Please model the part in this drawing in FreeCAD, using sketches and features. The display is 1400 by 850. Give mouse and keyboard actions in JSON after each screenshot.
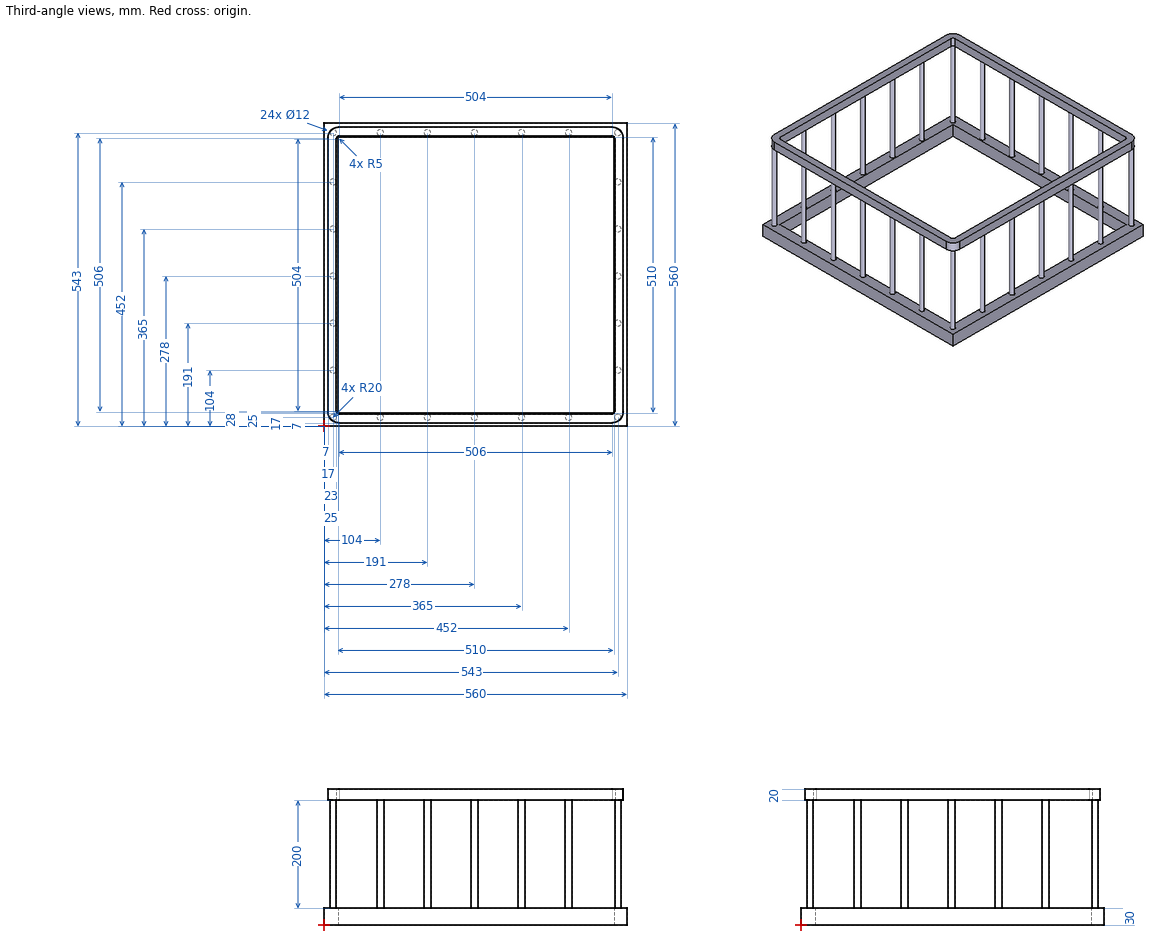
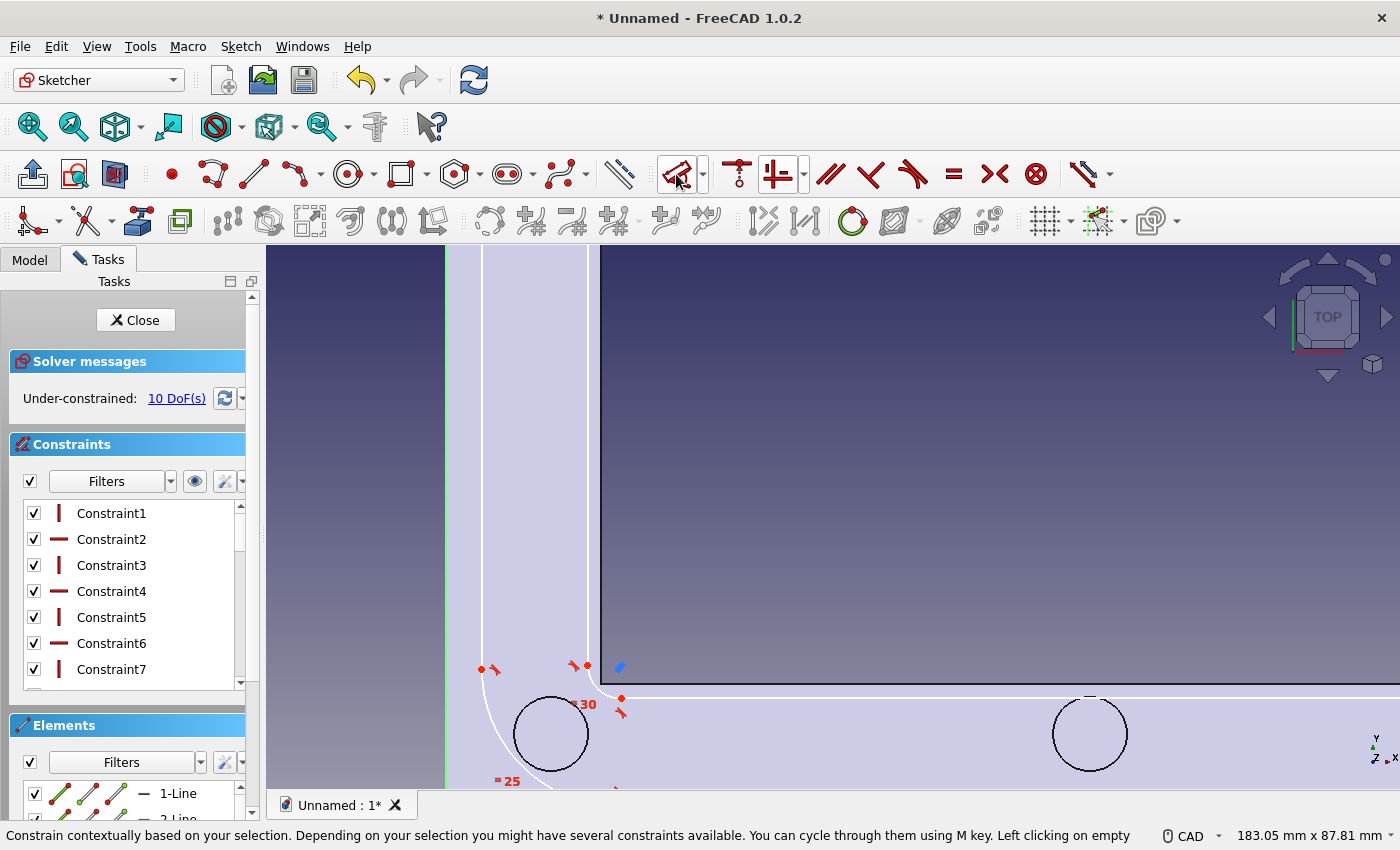
{"action": "scroll", "coordinate": [591, 690], "scroll_direction": "down", "scroll_amount": 11}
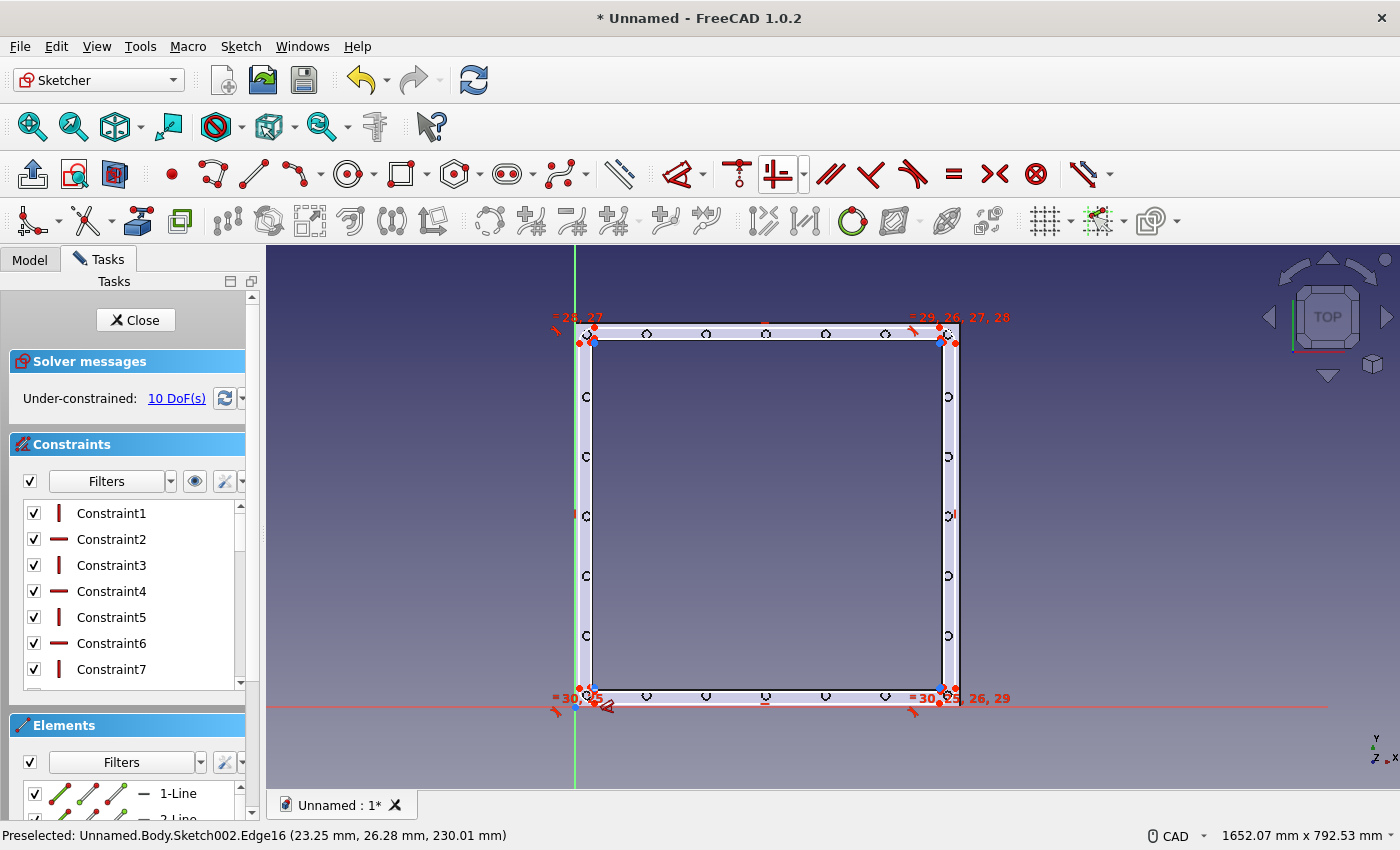
{"action": "scroll", "coordinate": [581, 695], "scroll_direction": "up", "scroll_amount": 6}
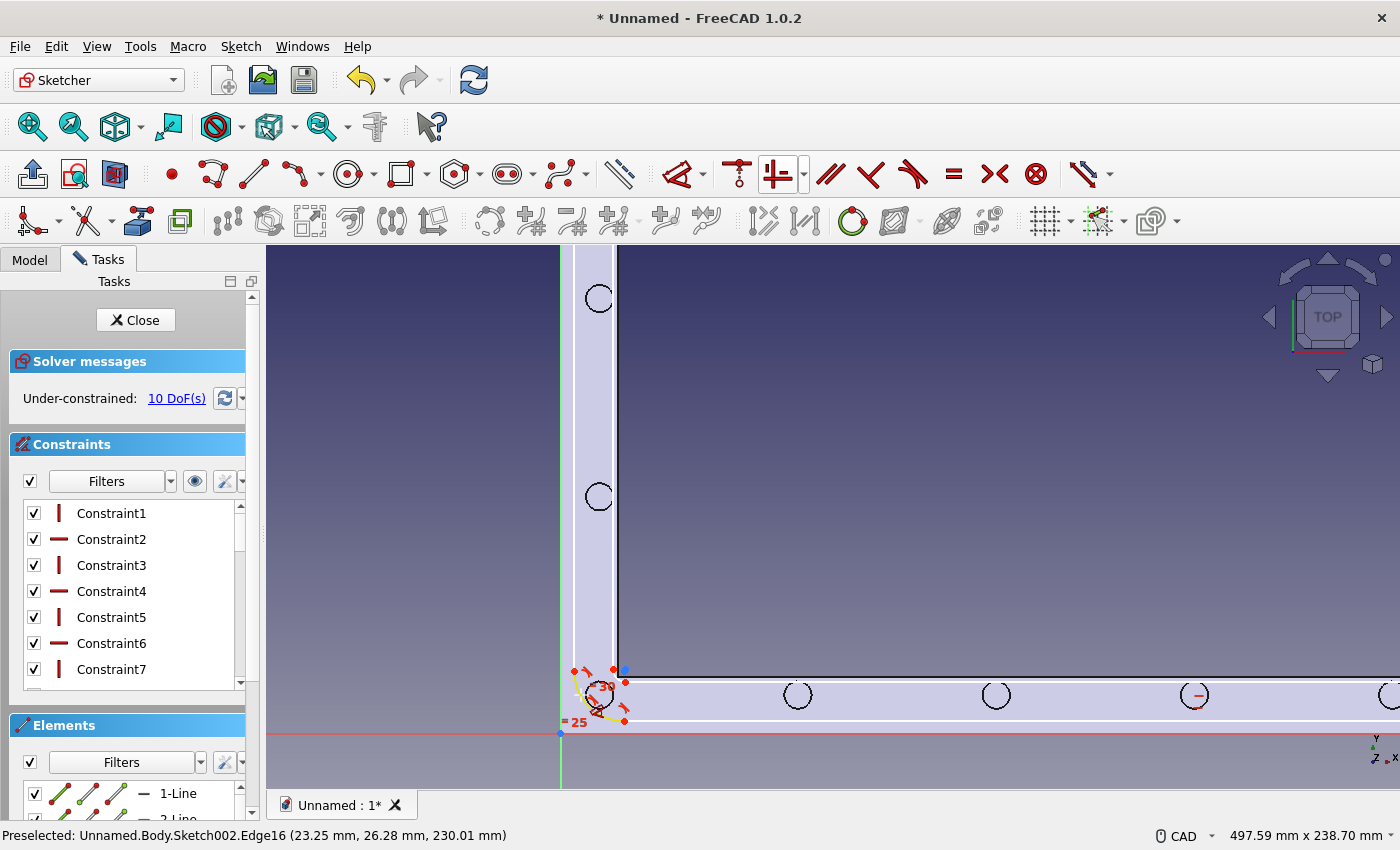
{"action": "left_click", "coordinate": [580, 694]}
{"action": "left_click", "coordinate": [543, 669]}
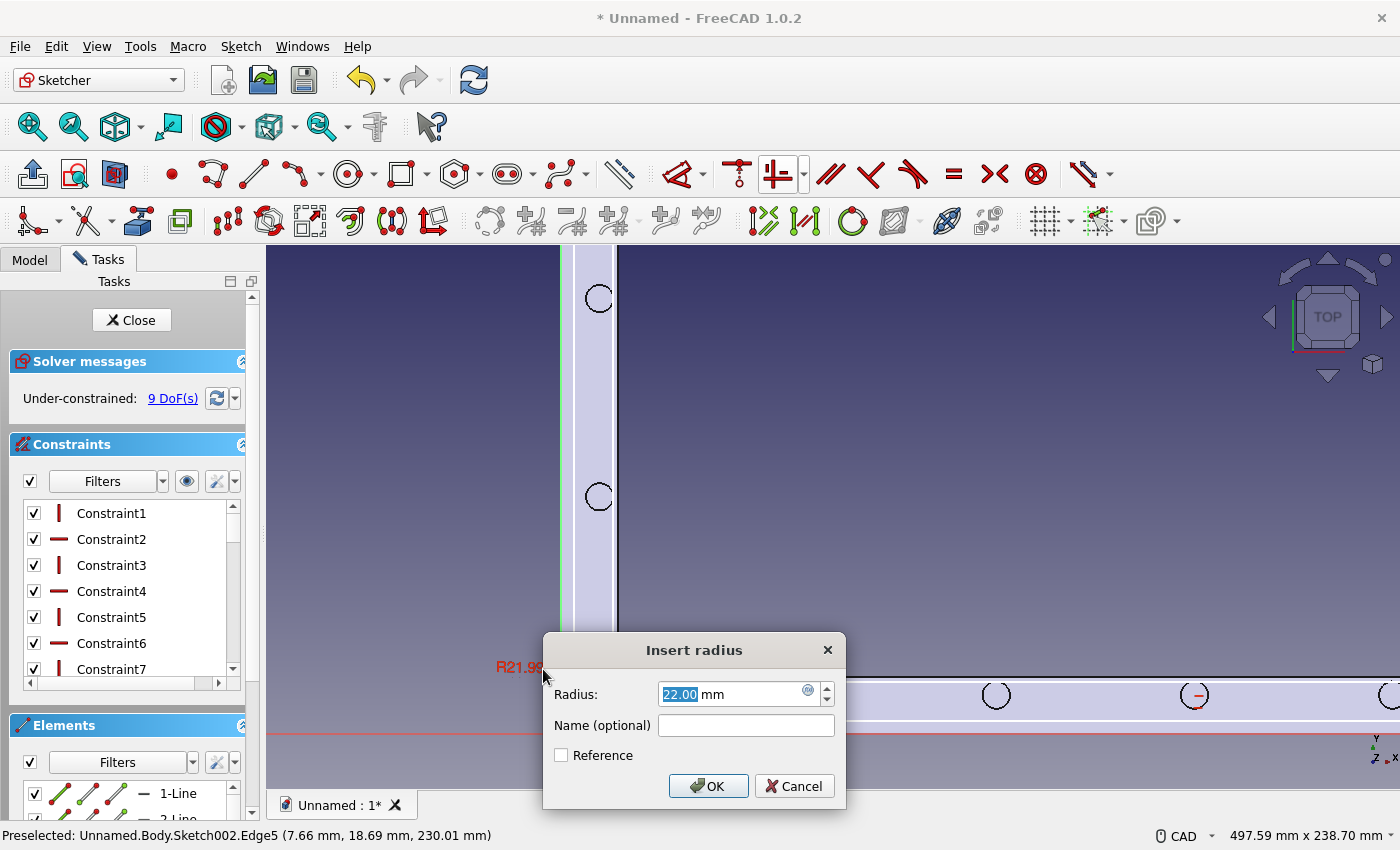
{"action": "type", "text": "20"}
{"action": "key", "text": "Return"}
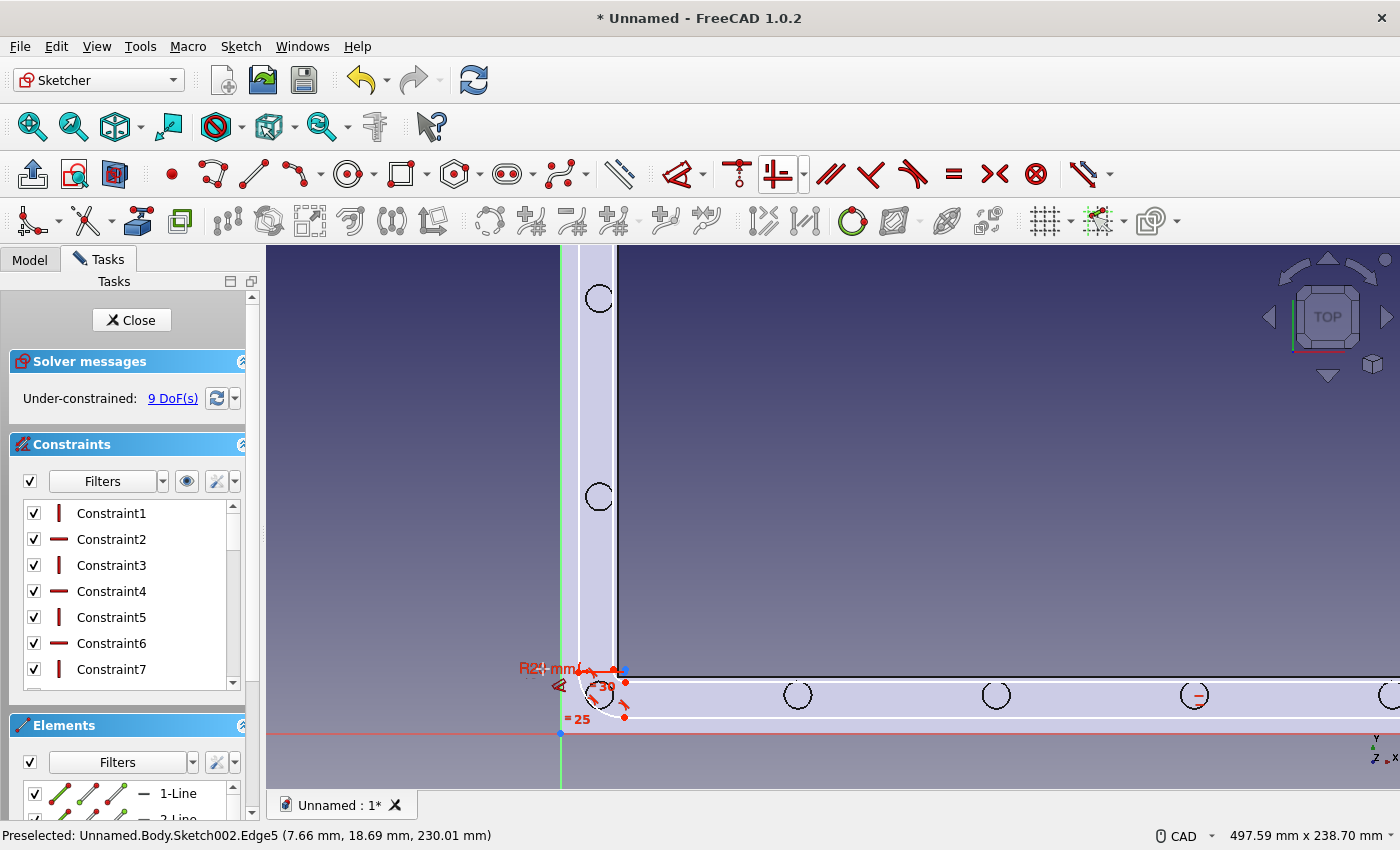
{"action": "scroll", "coordinate": [581, 695], "scroll_direction": "down", "scroll_amount": 6}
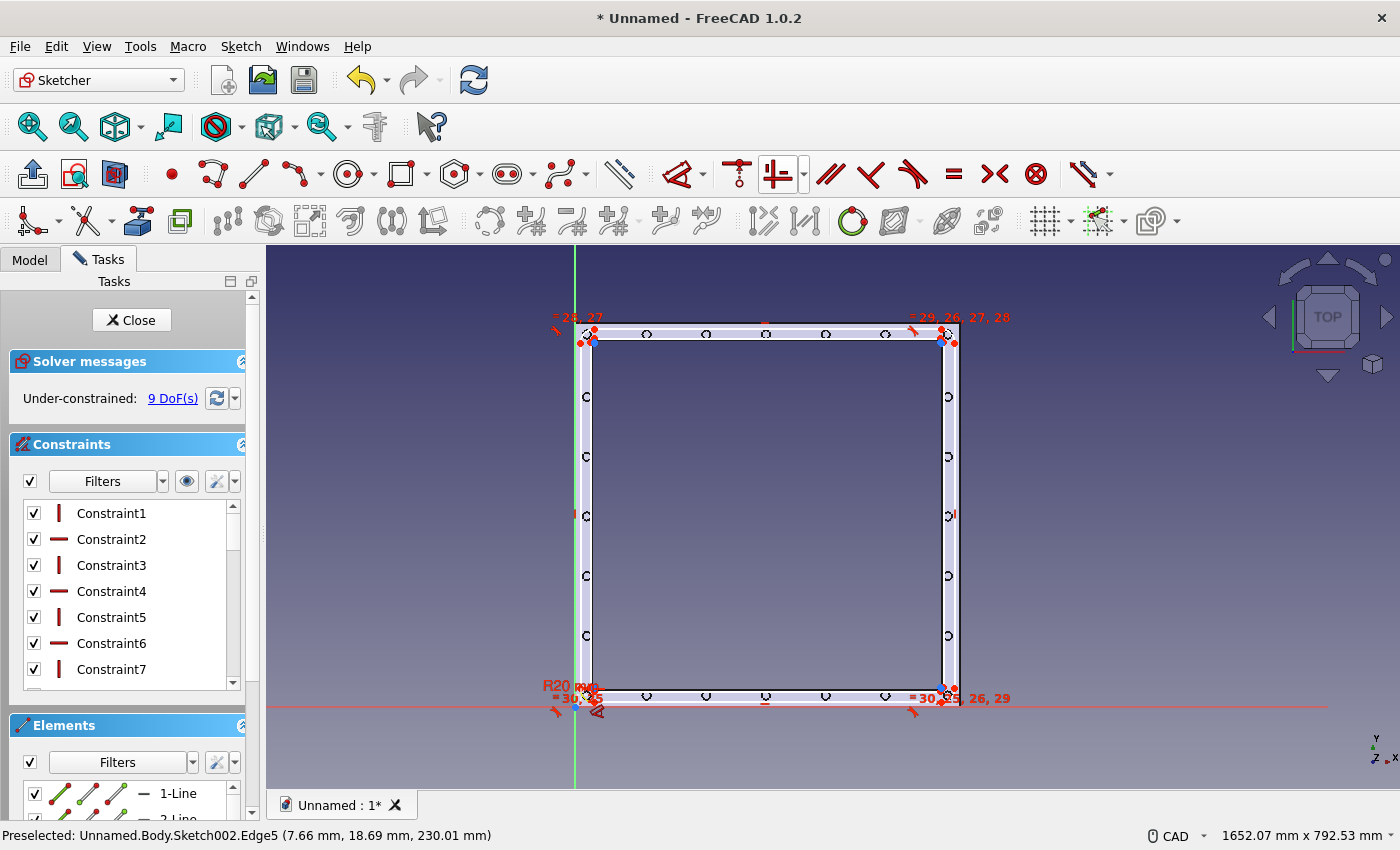
{"action": "scroll", "coordinate": [592, 340], "scroll_direction": "up", "scroll_amount": 13}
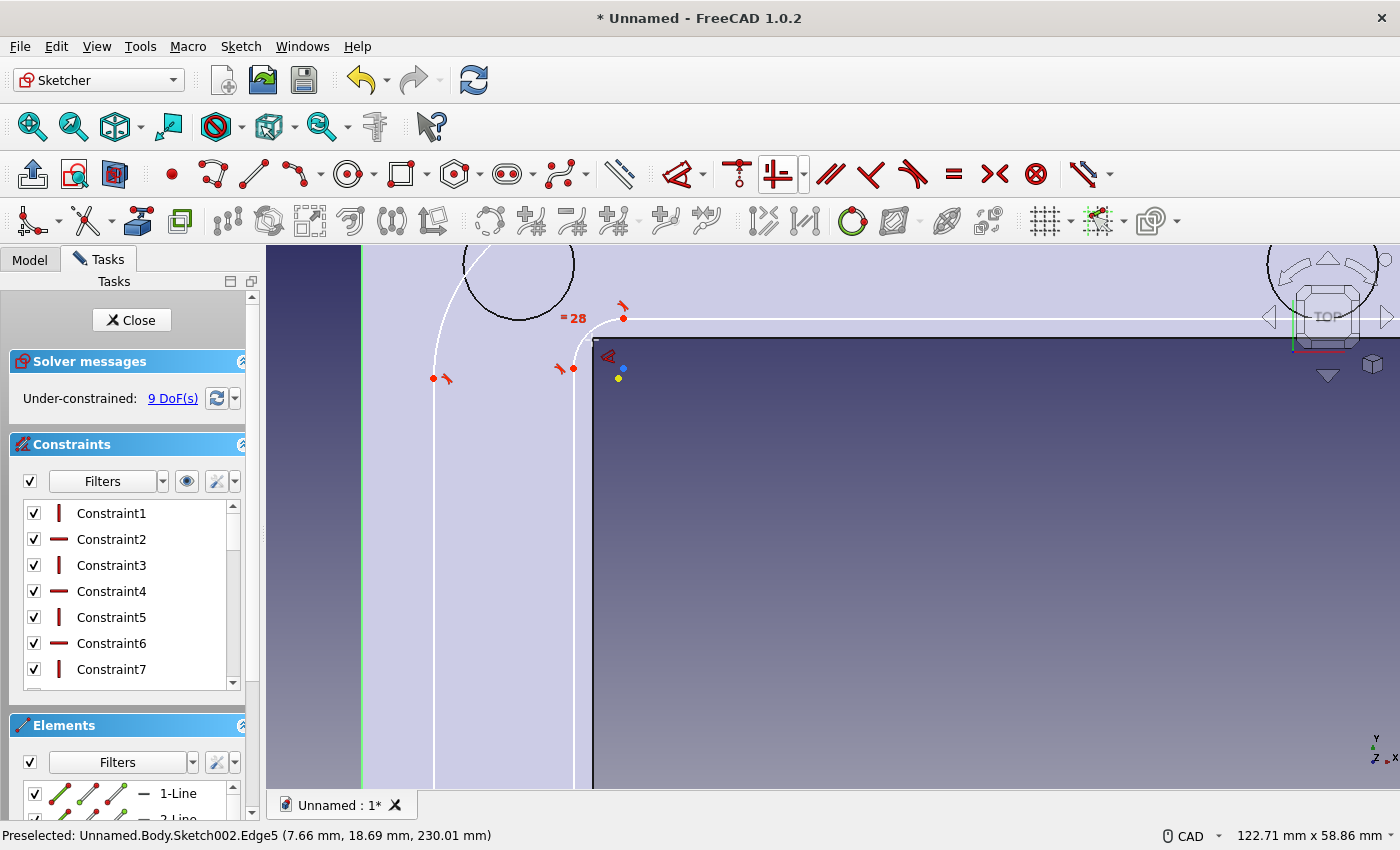
{"action": "left_click", "coordinate": [588, 333]}
{"action": "left_click", "coordinate": [565, 310]}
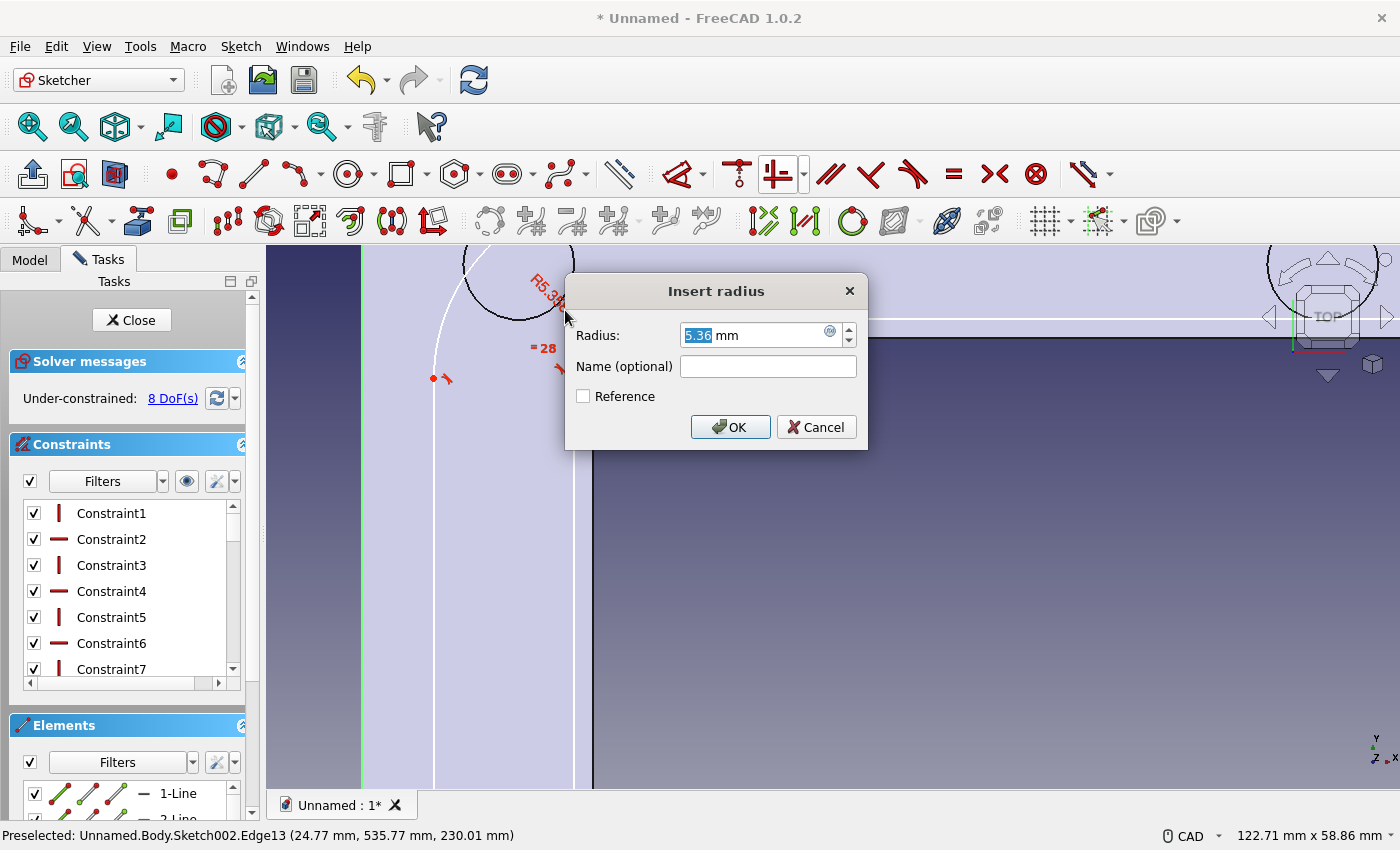
{"action": "type", "text": "5"}
{"action": "key", "text": "Return"}